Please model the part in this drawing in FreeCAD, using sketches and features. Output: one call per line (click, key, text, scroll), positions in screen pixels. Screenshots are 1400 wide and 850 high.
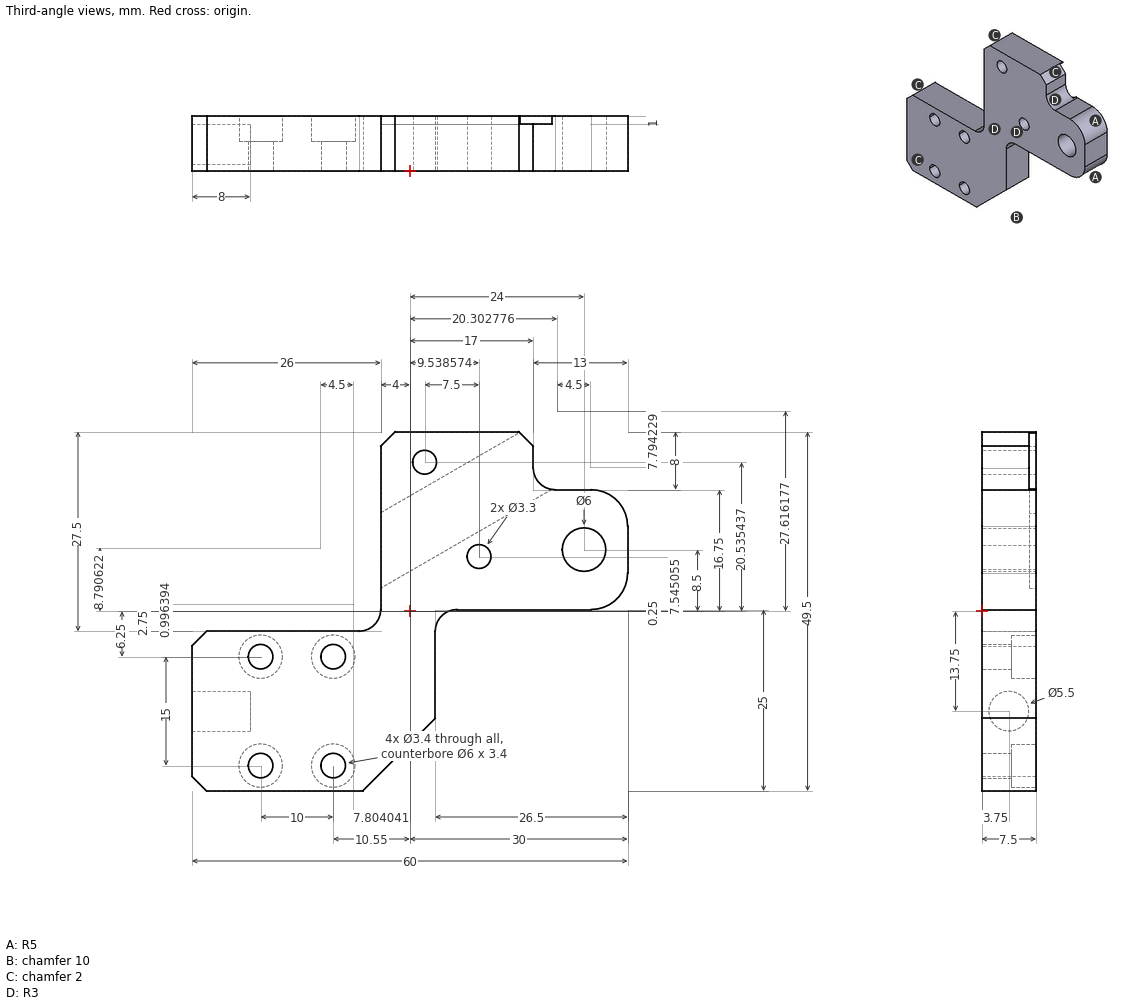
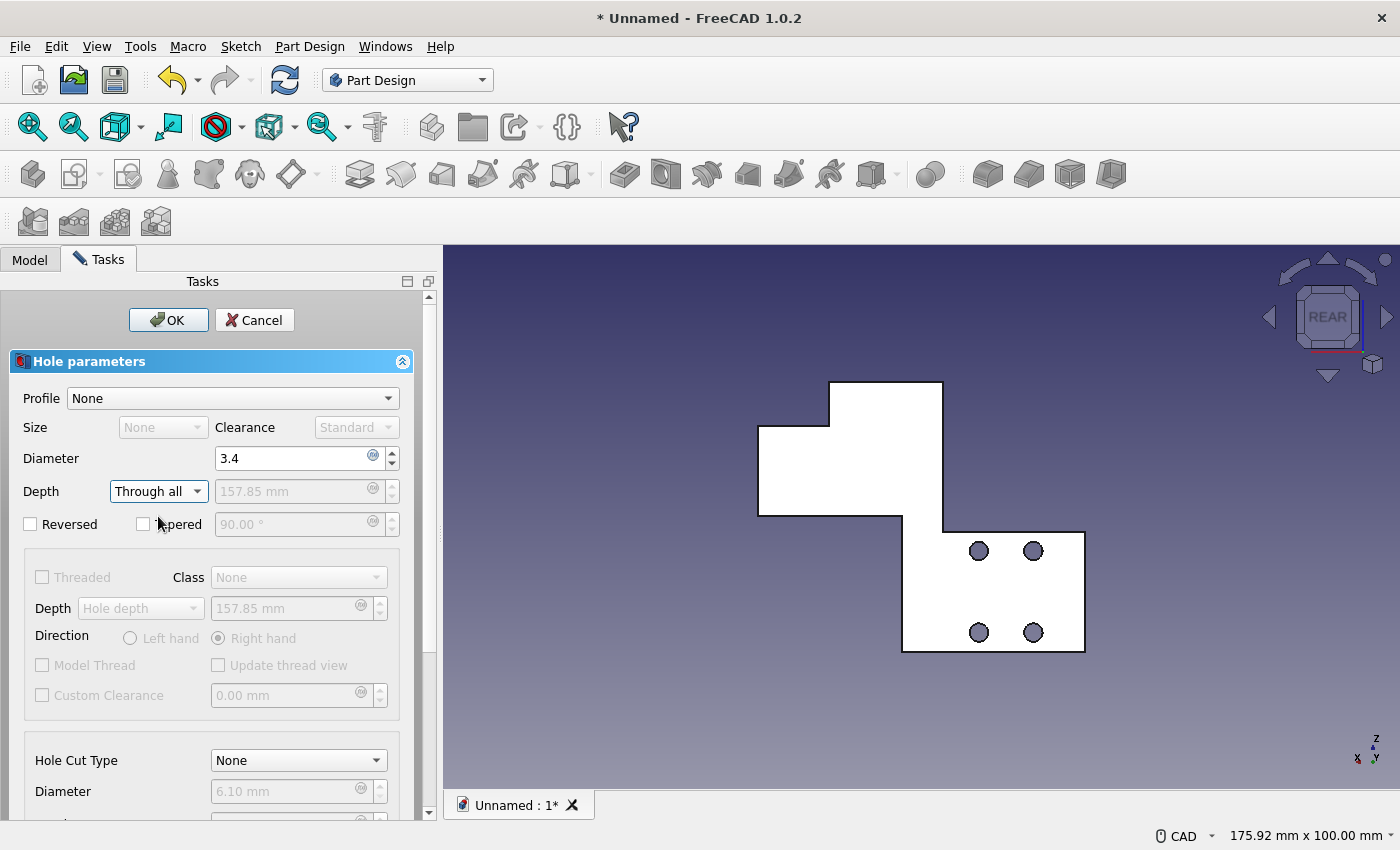
click(300, 760)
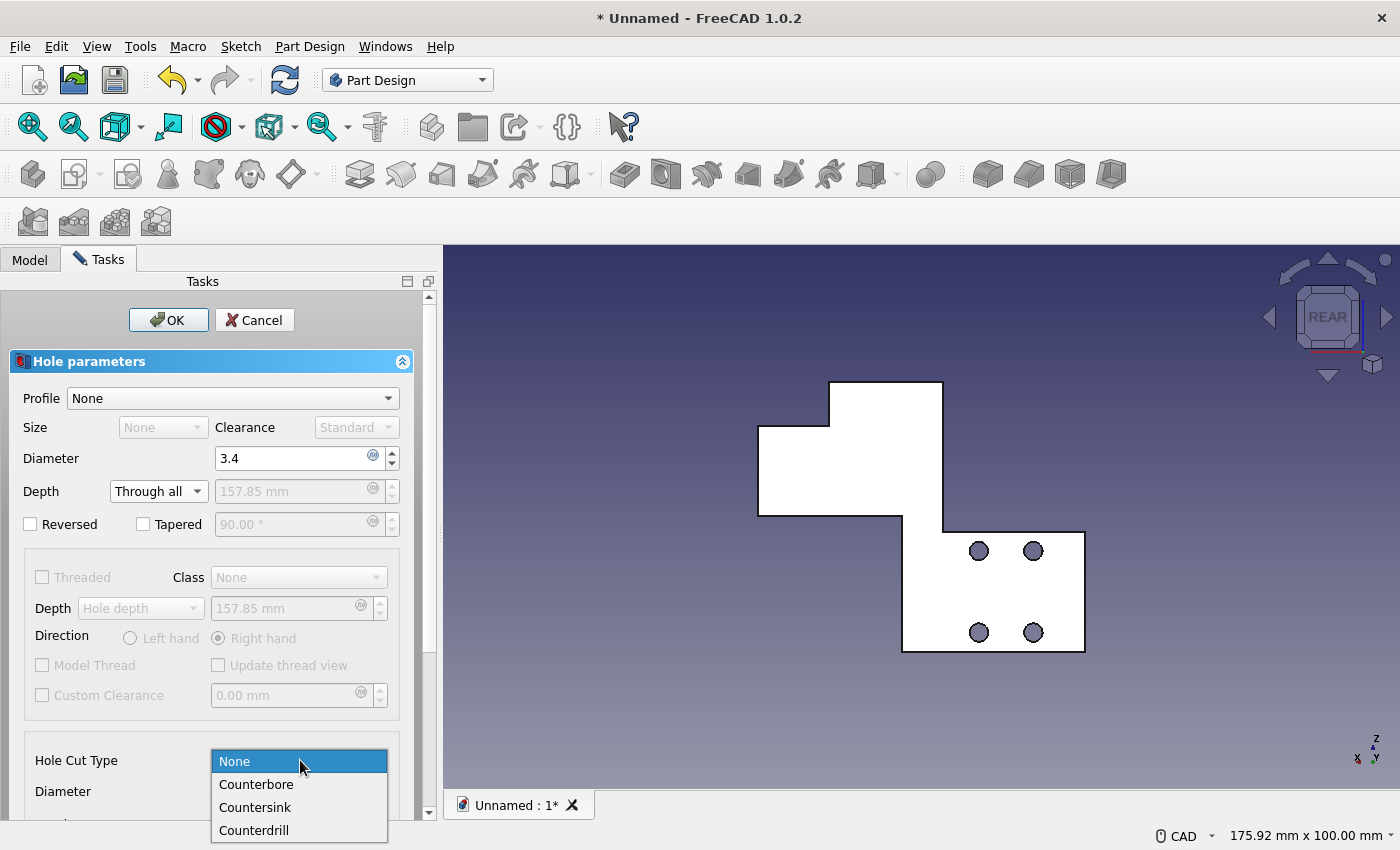
click(298, 784)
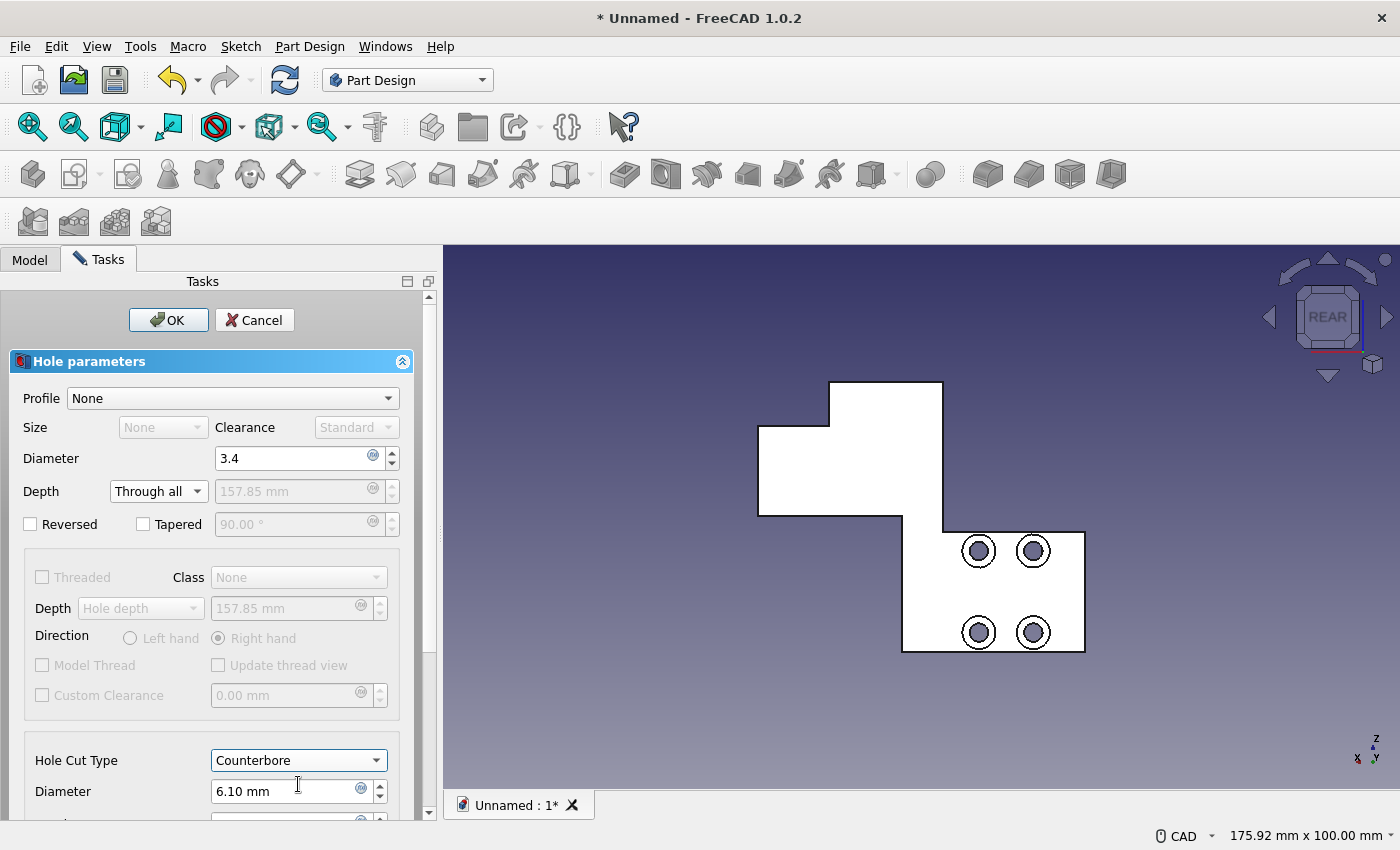
triple_click(292, 792)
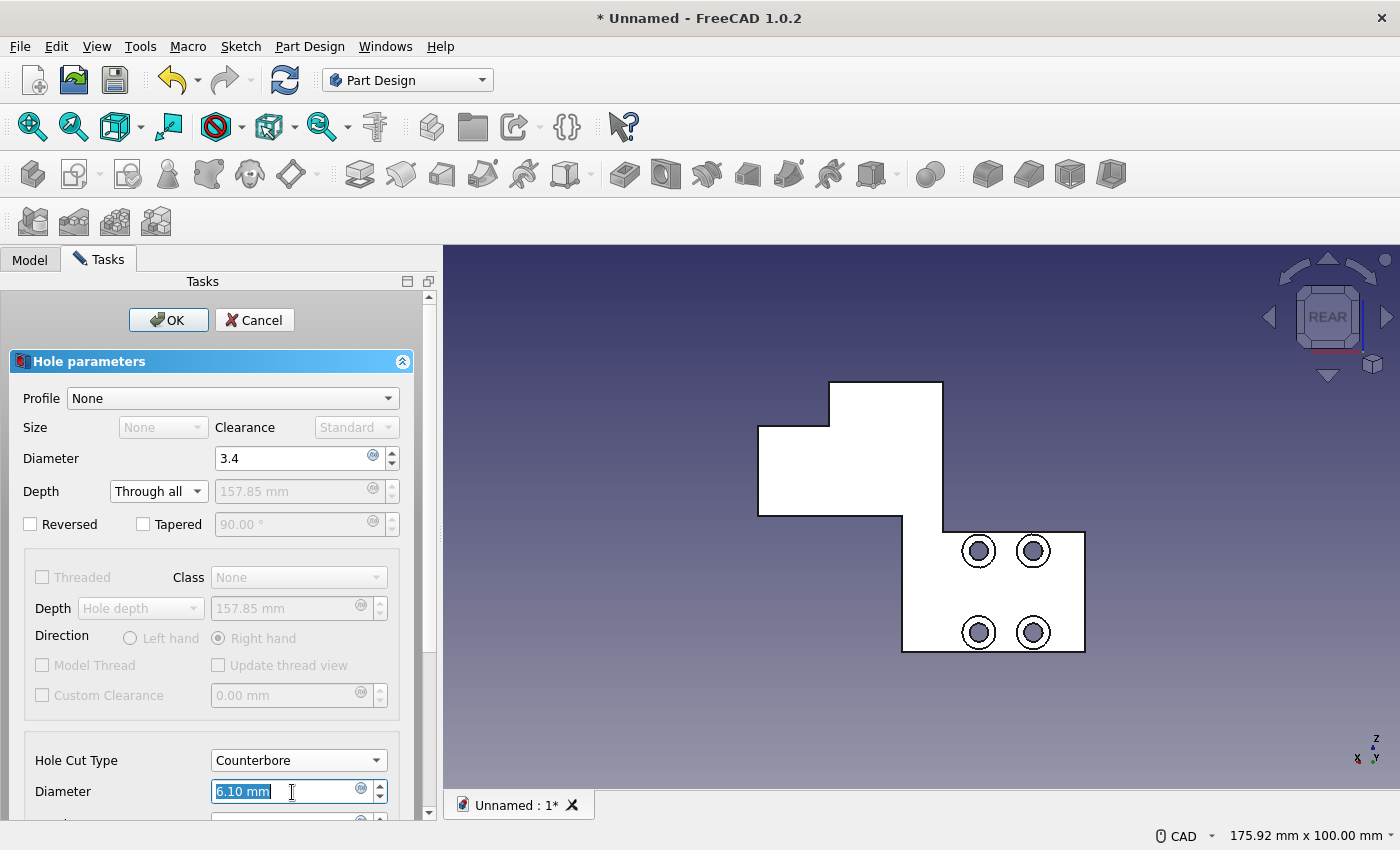
text(6)
key(Tab)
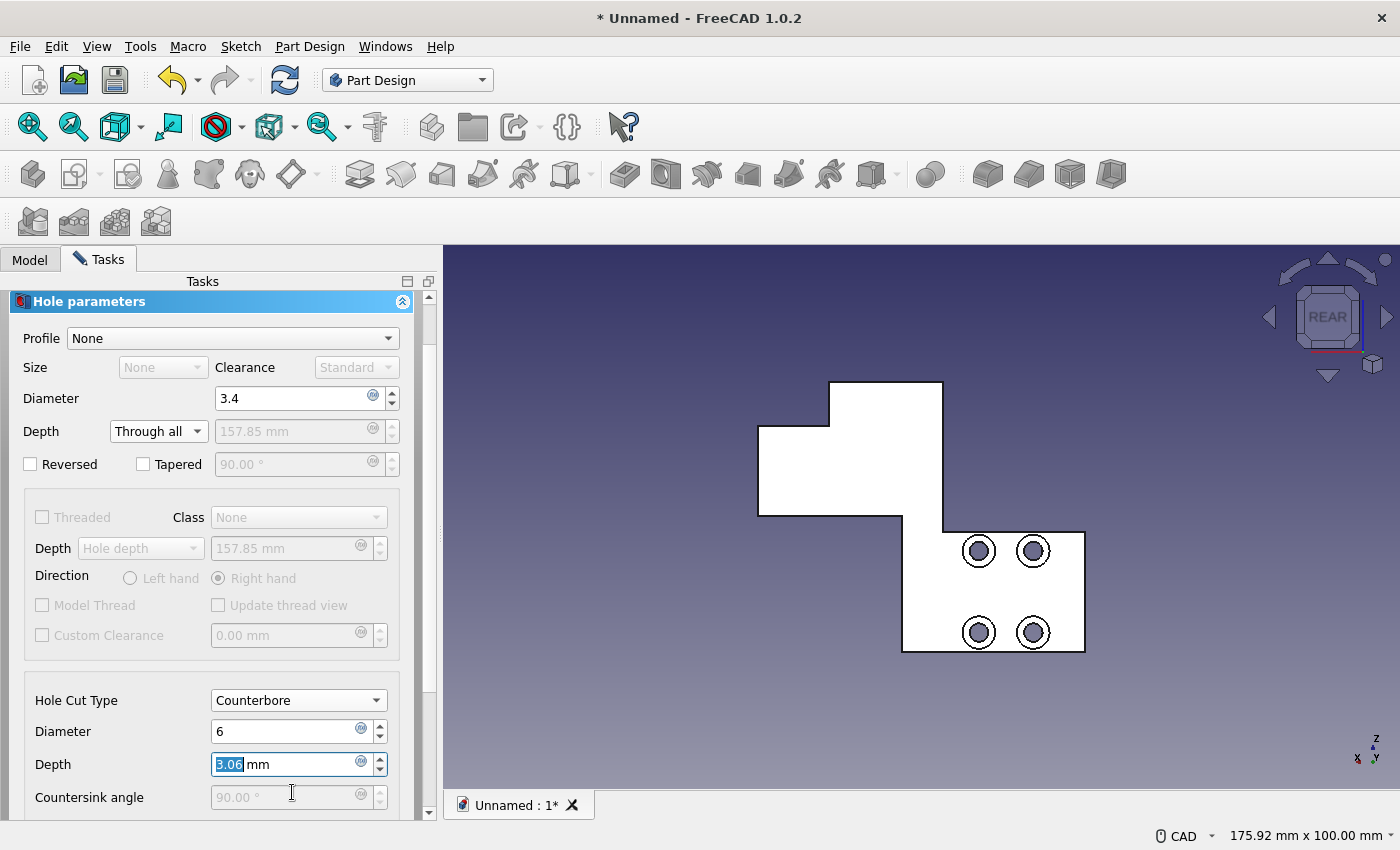
text(3.4)
key(Tab)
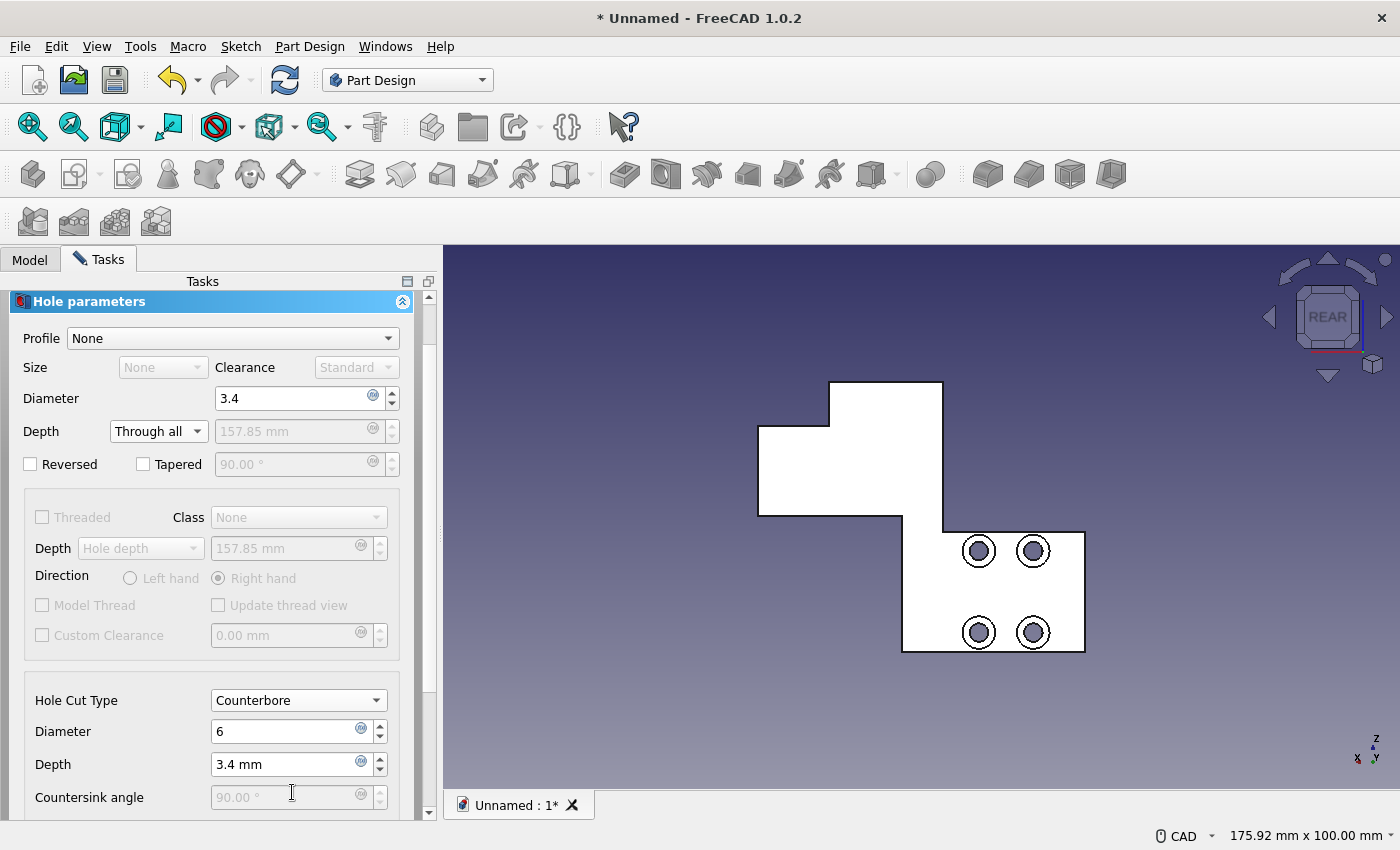
scroll(429, 556, up, 2)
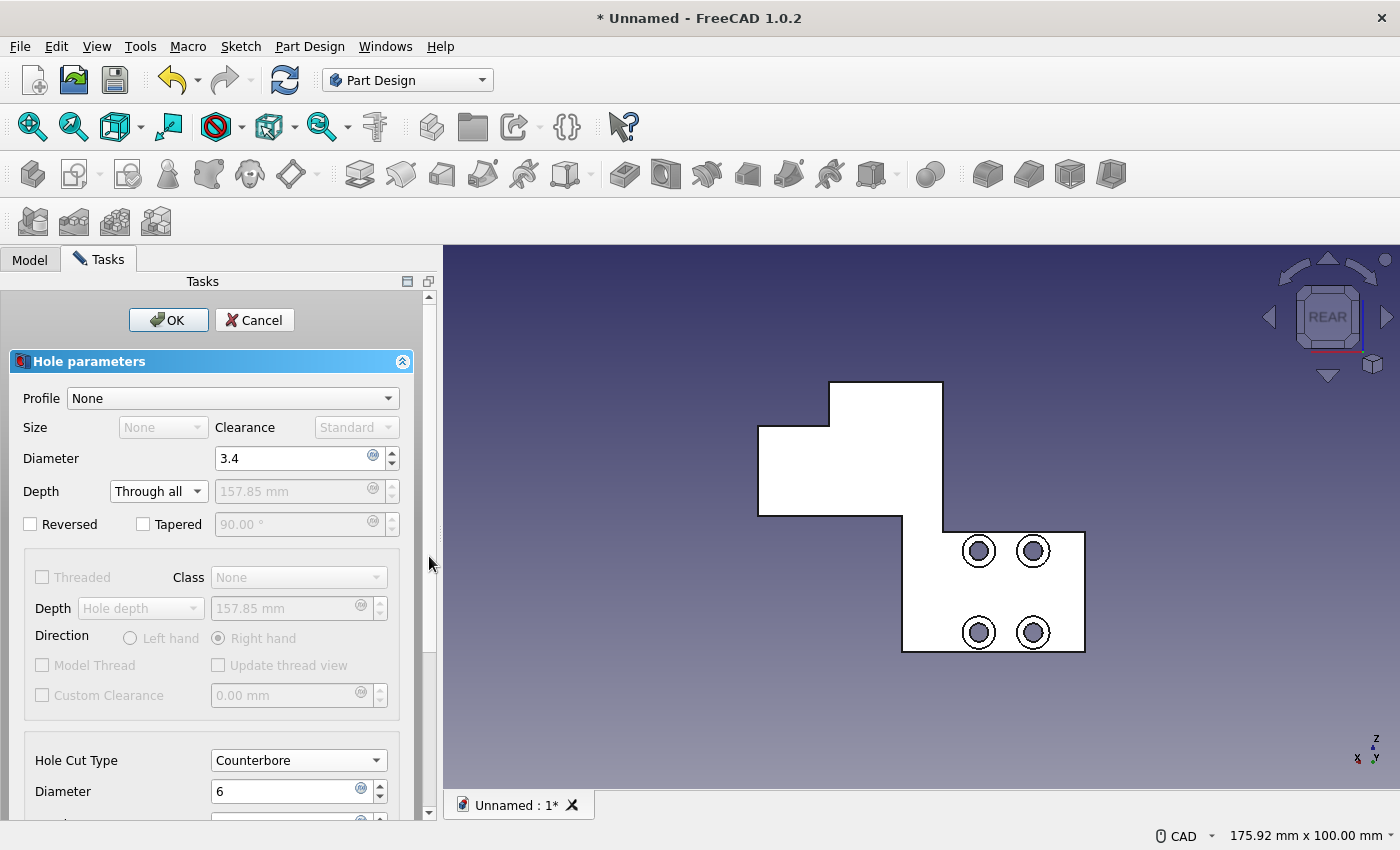
click(169, 320)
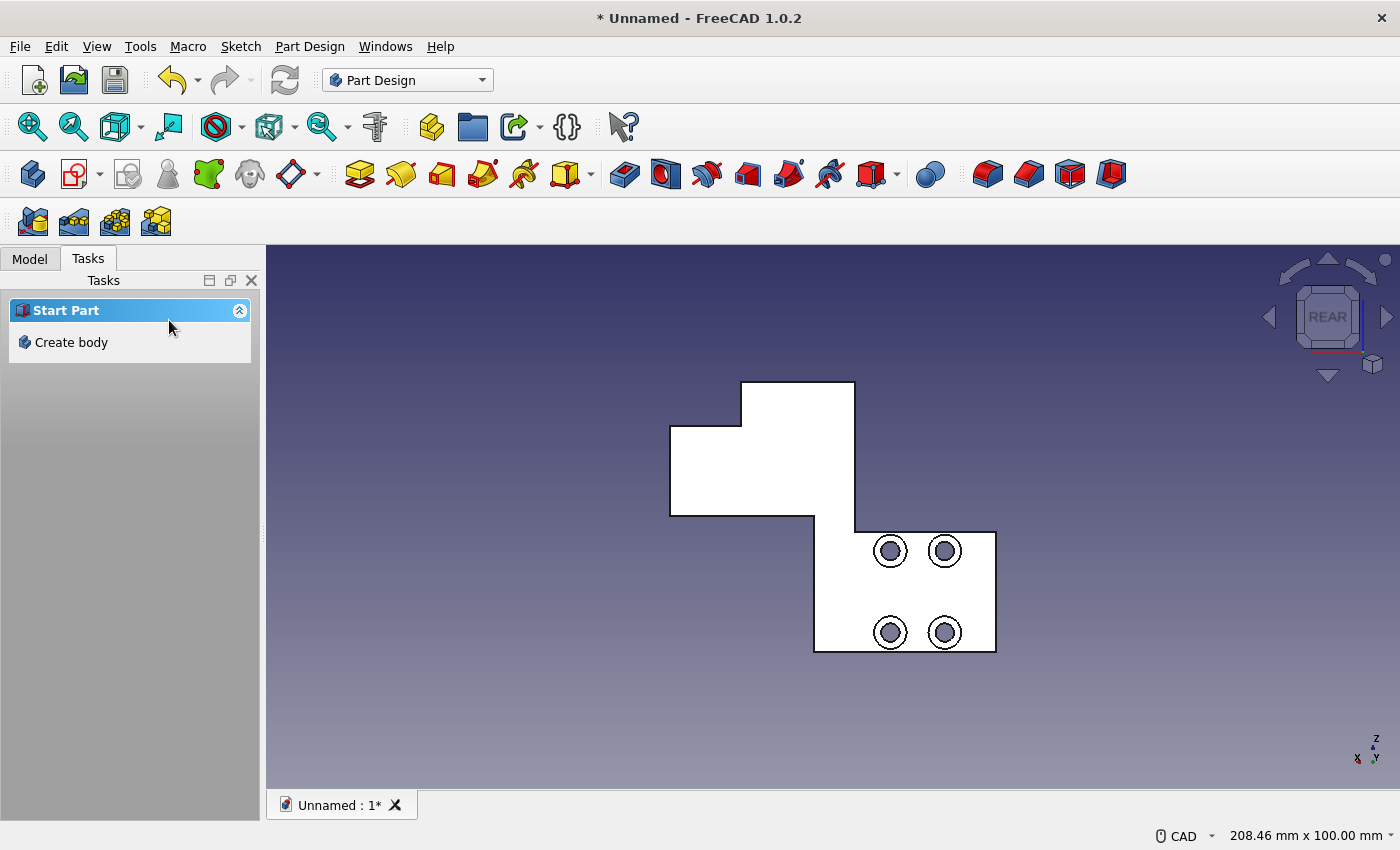
click(786, 439)